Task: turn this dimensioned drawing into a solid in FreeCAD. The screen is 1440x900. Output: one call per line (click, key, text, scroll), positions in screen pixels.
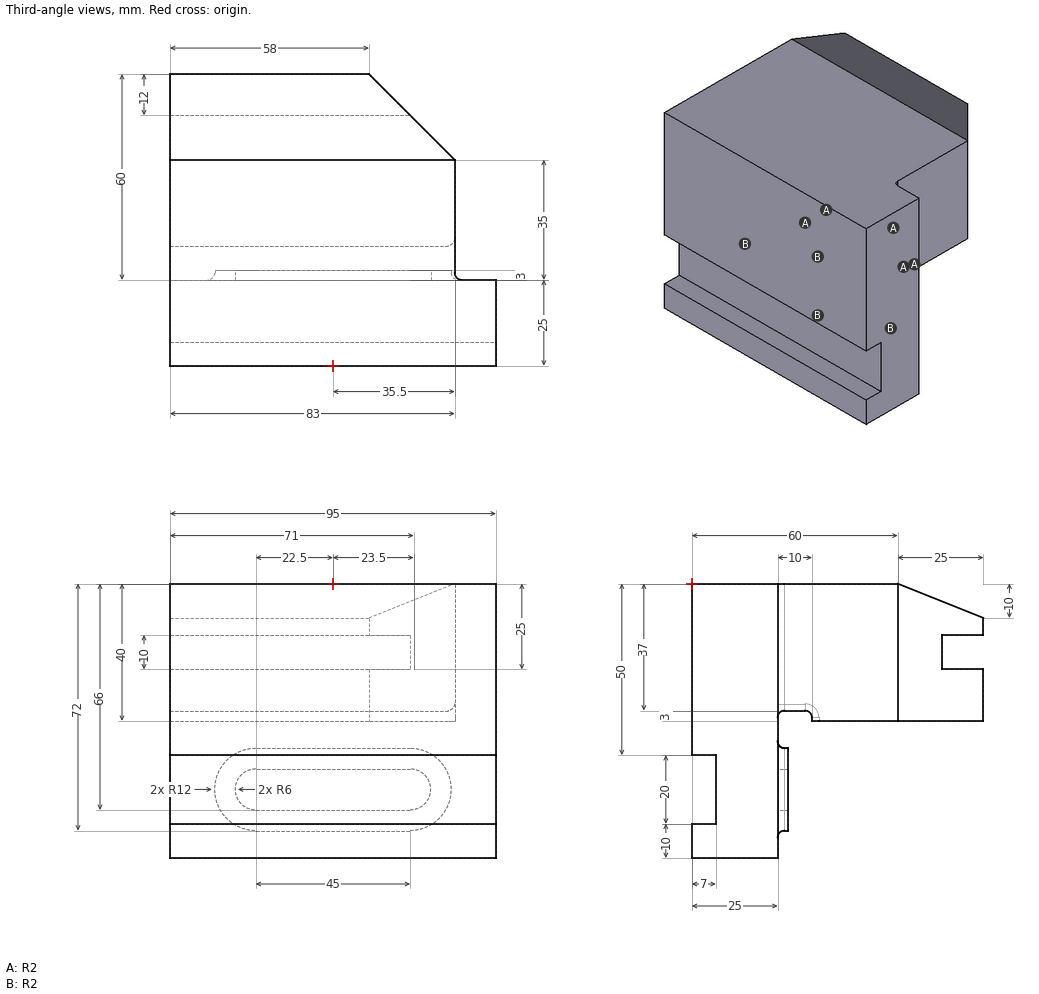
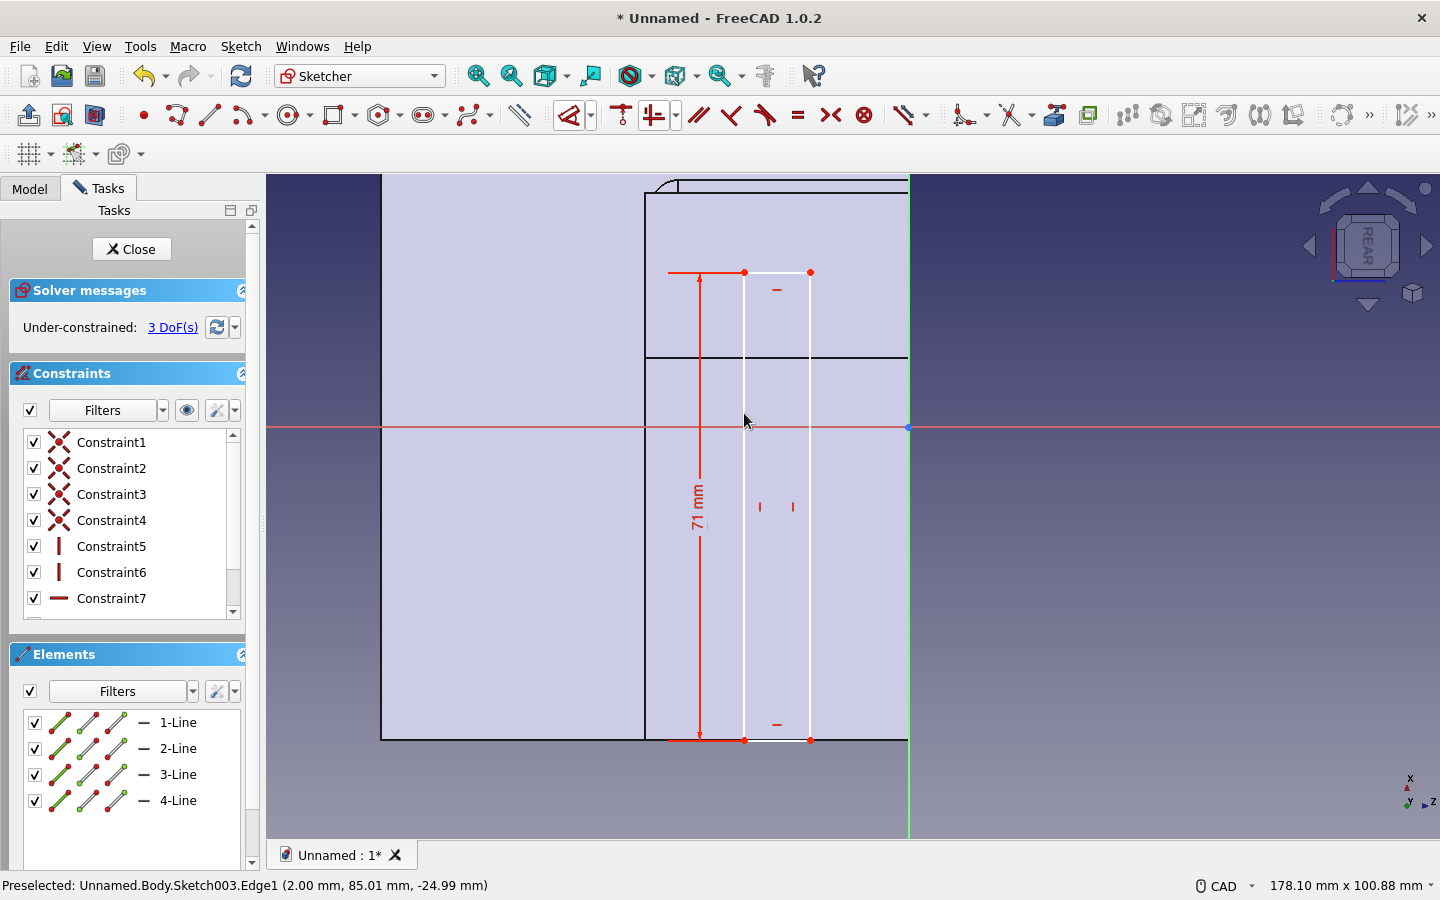
click(764, 741)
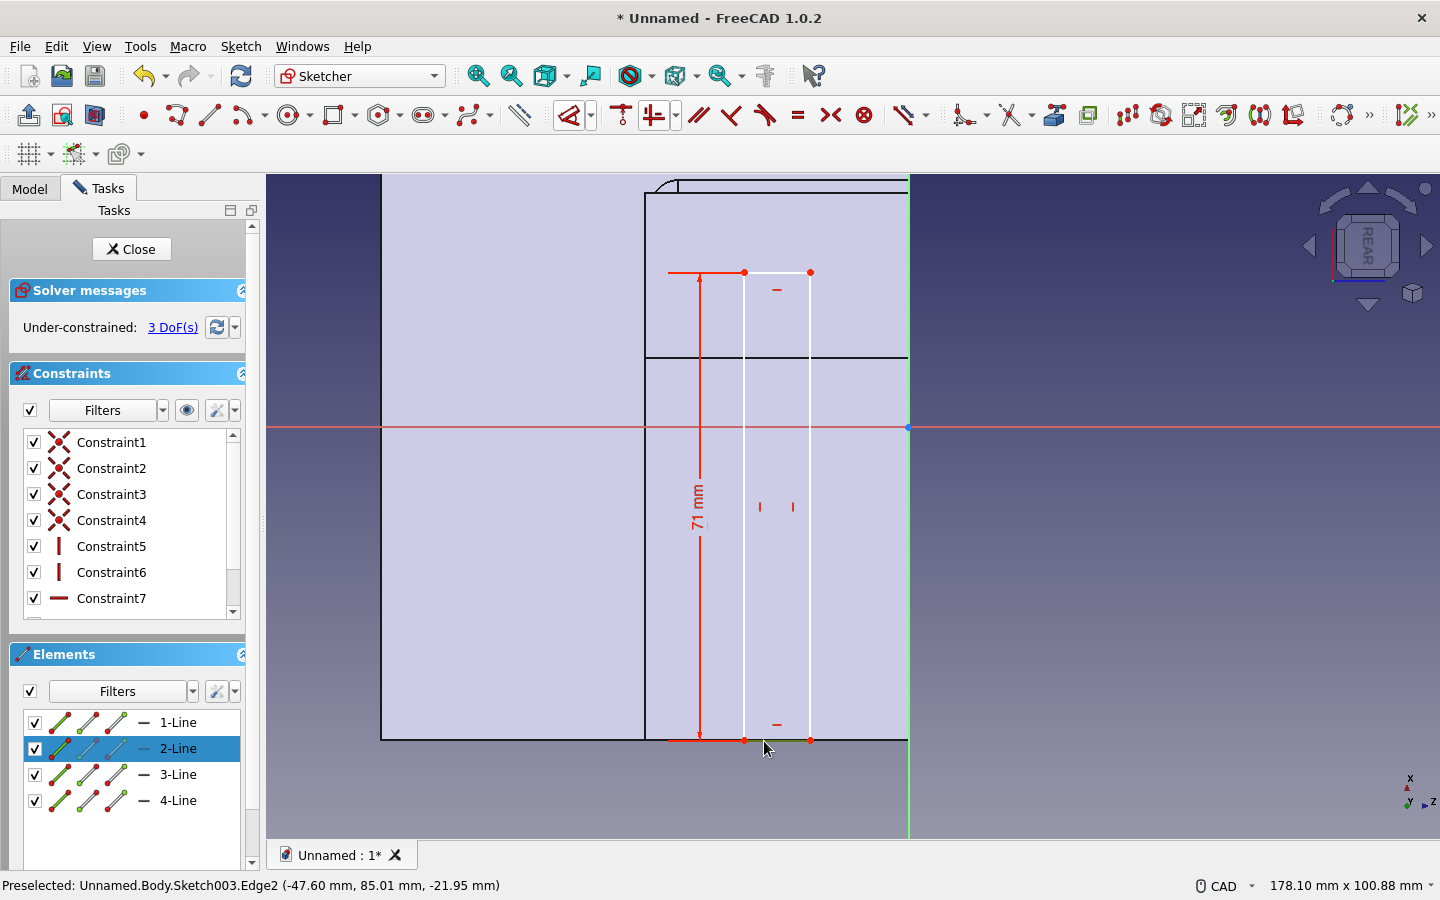
key(l)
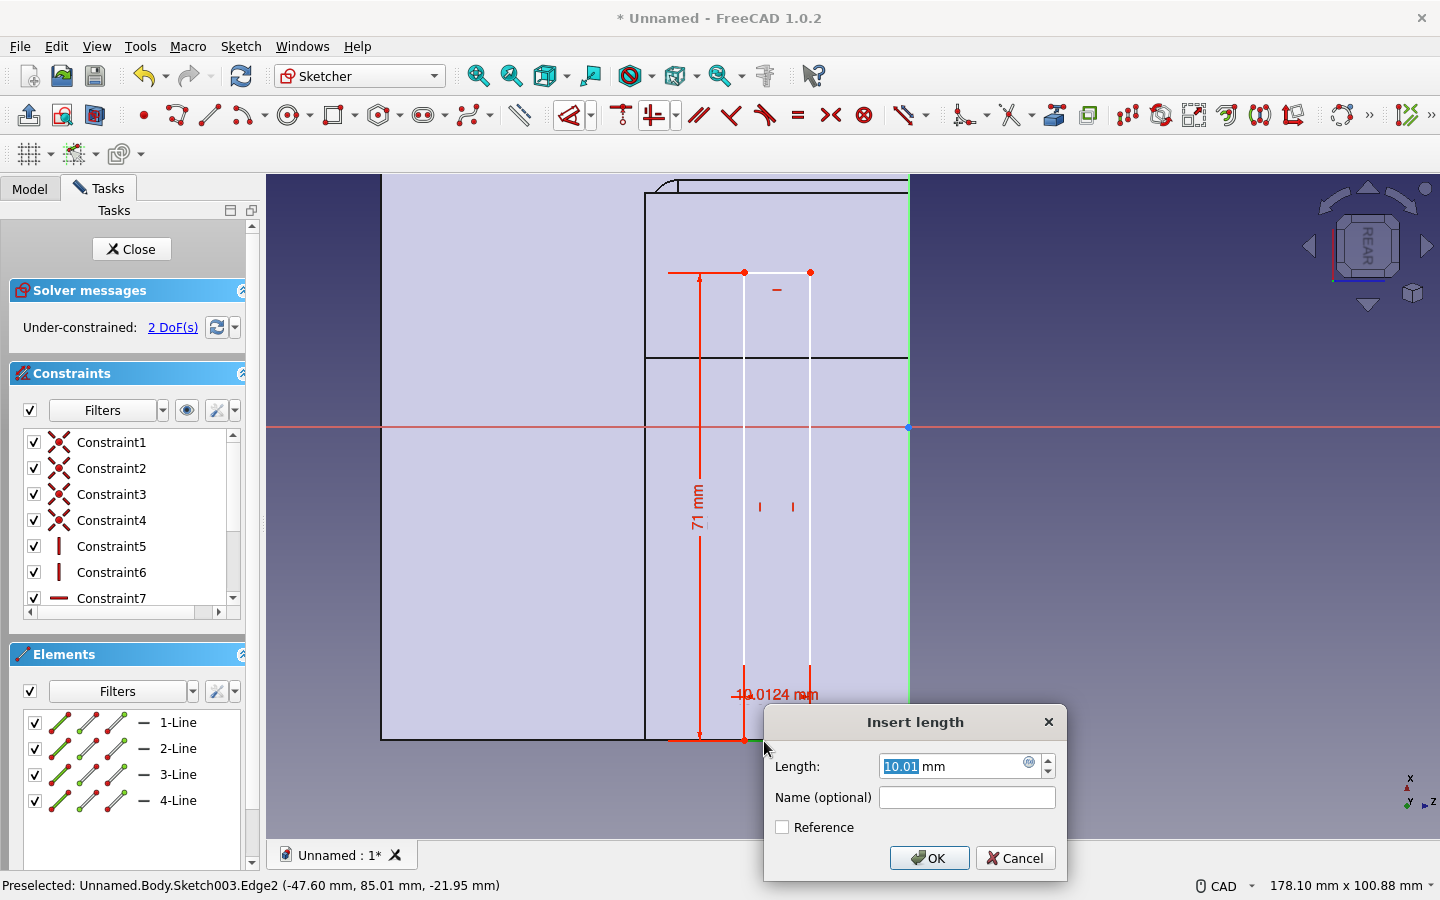
text(10)
key(Return)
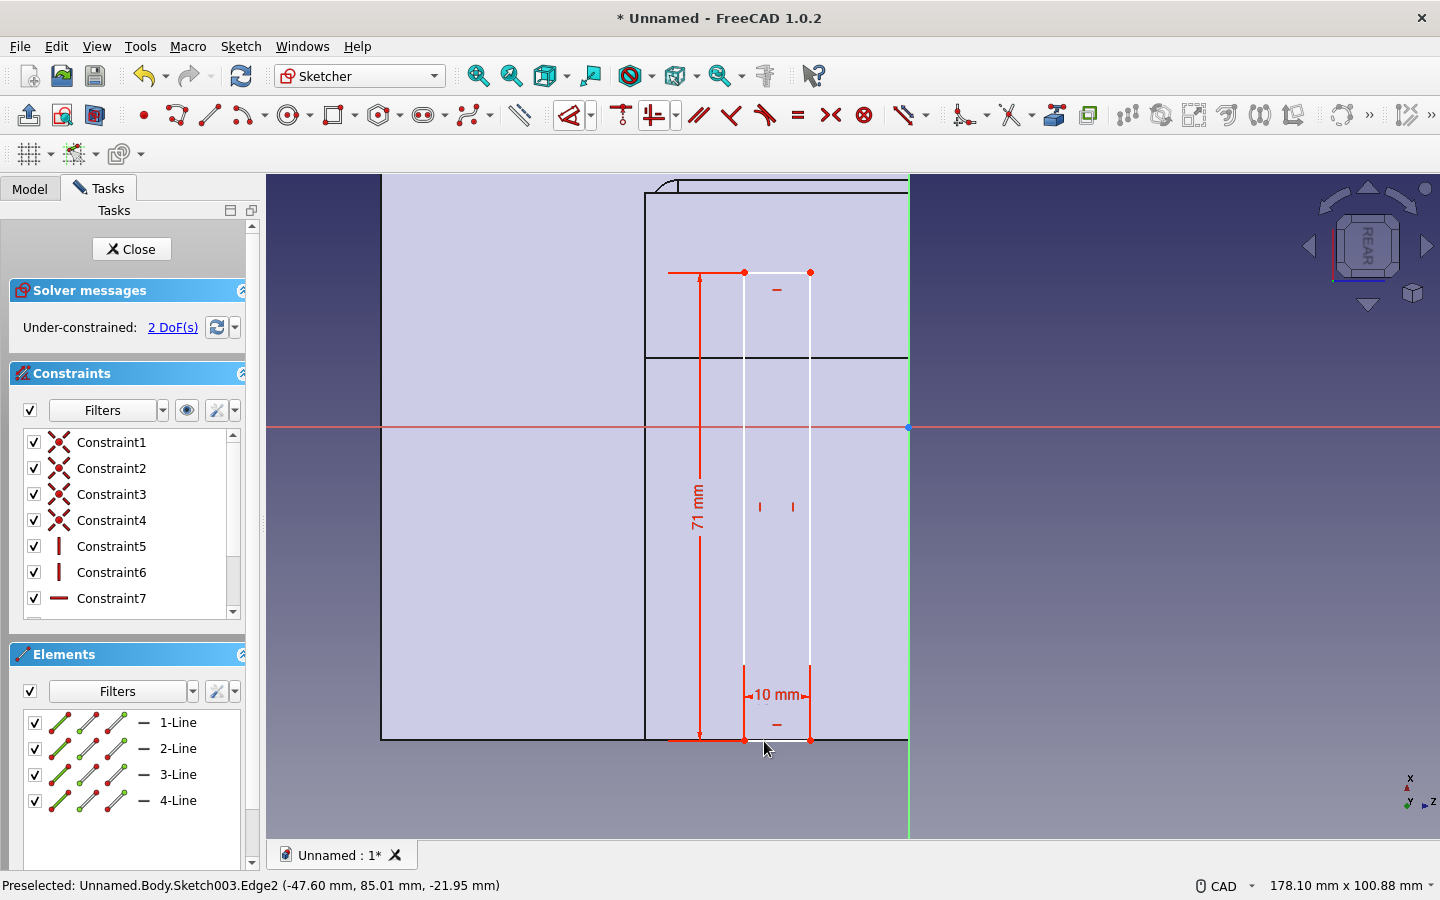
click(744, 273)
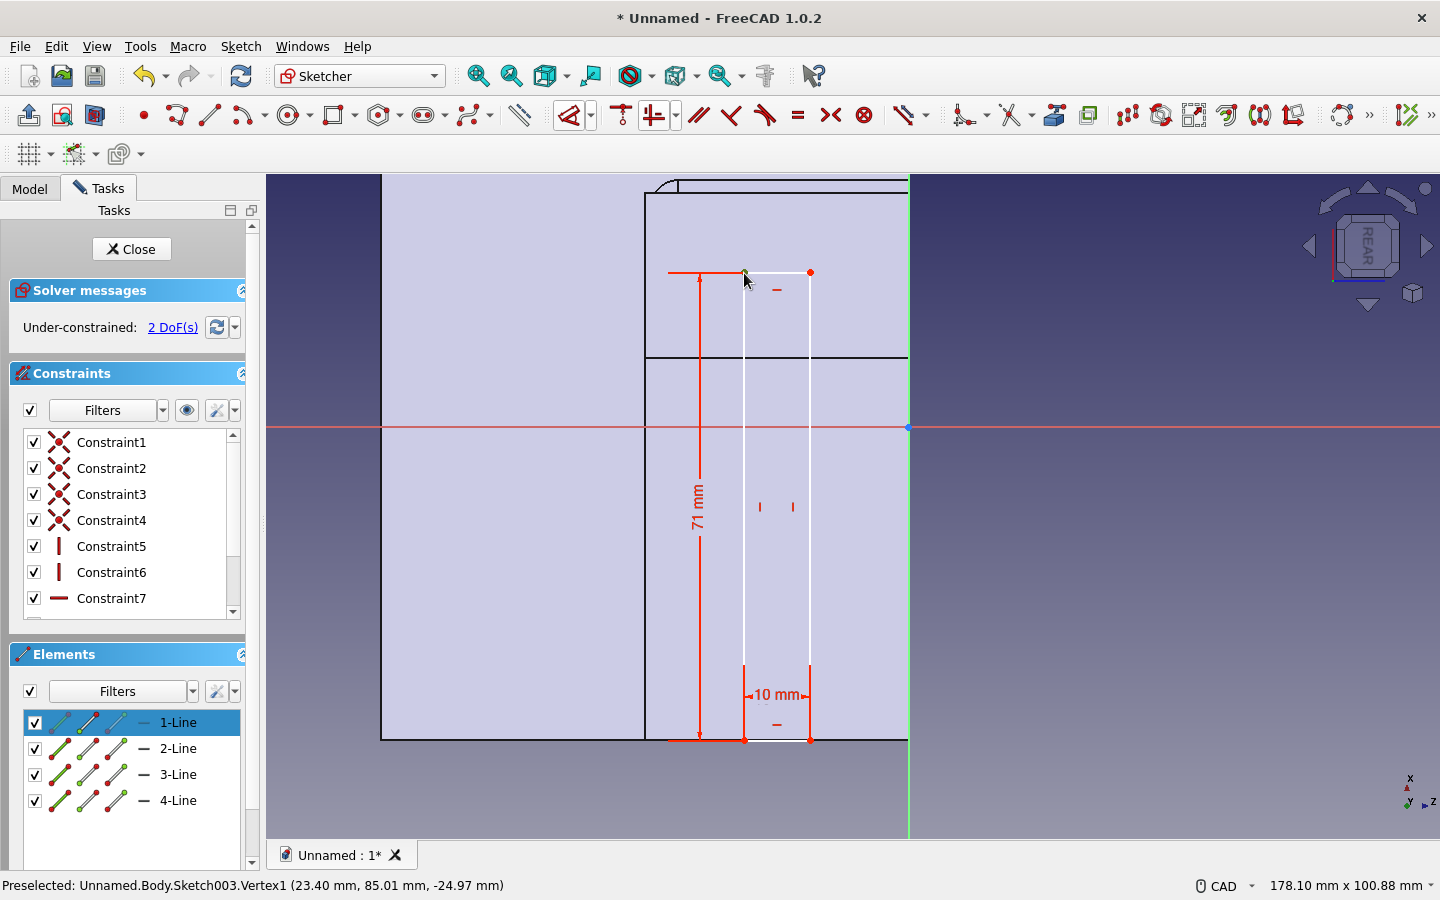
click(590, 116)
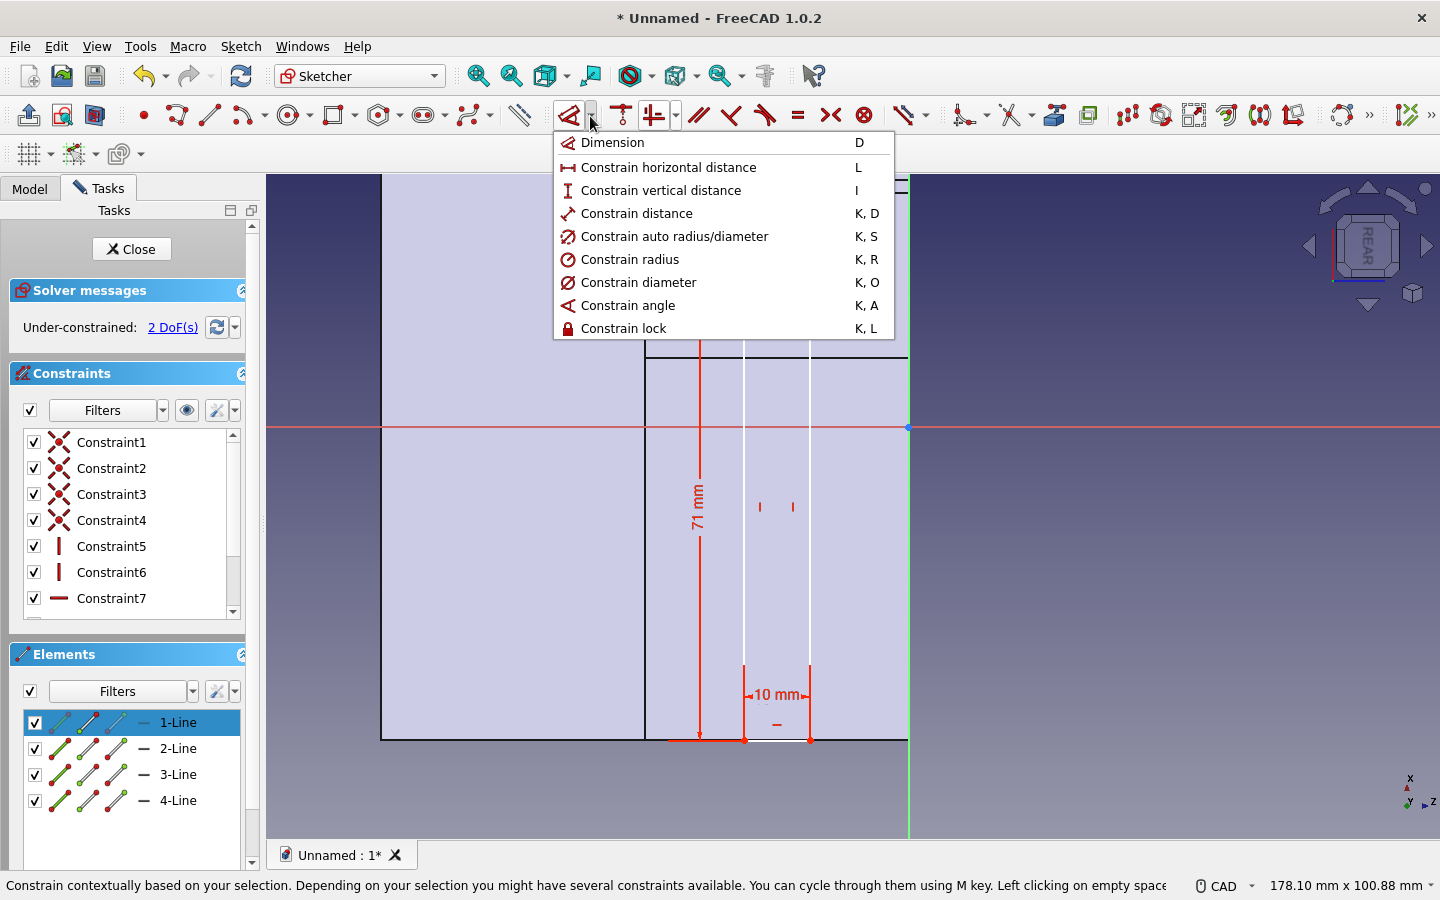
click(724, 168)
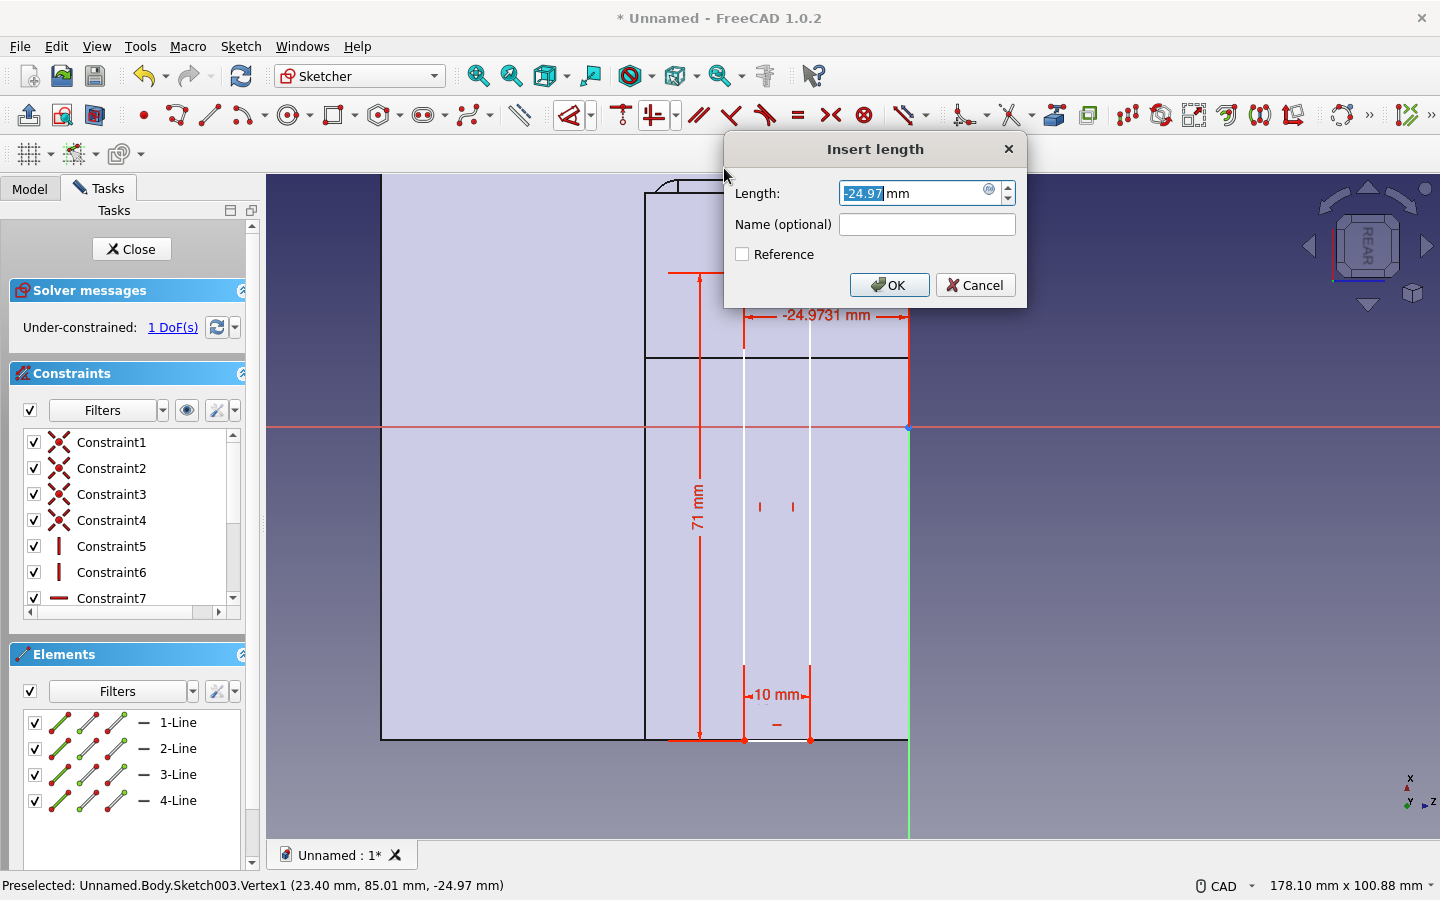
text(-25)
key(Return)